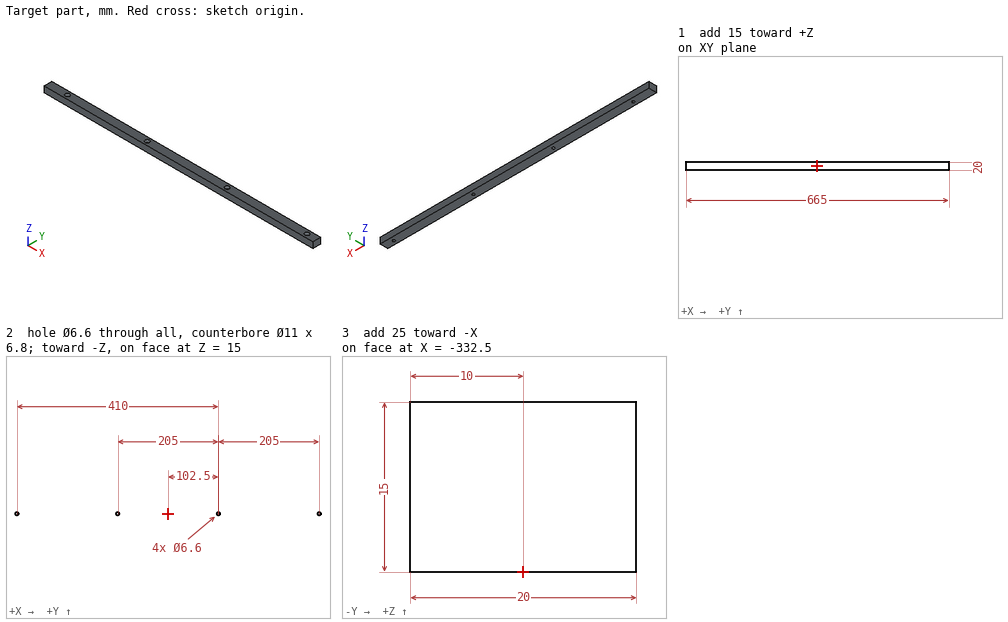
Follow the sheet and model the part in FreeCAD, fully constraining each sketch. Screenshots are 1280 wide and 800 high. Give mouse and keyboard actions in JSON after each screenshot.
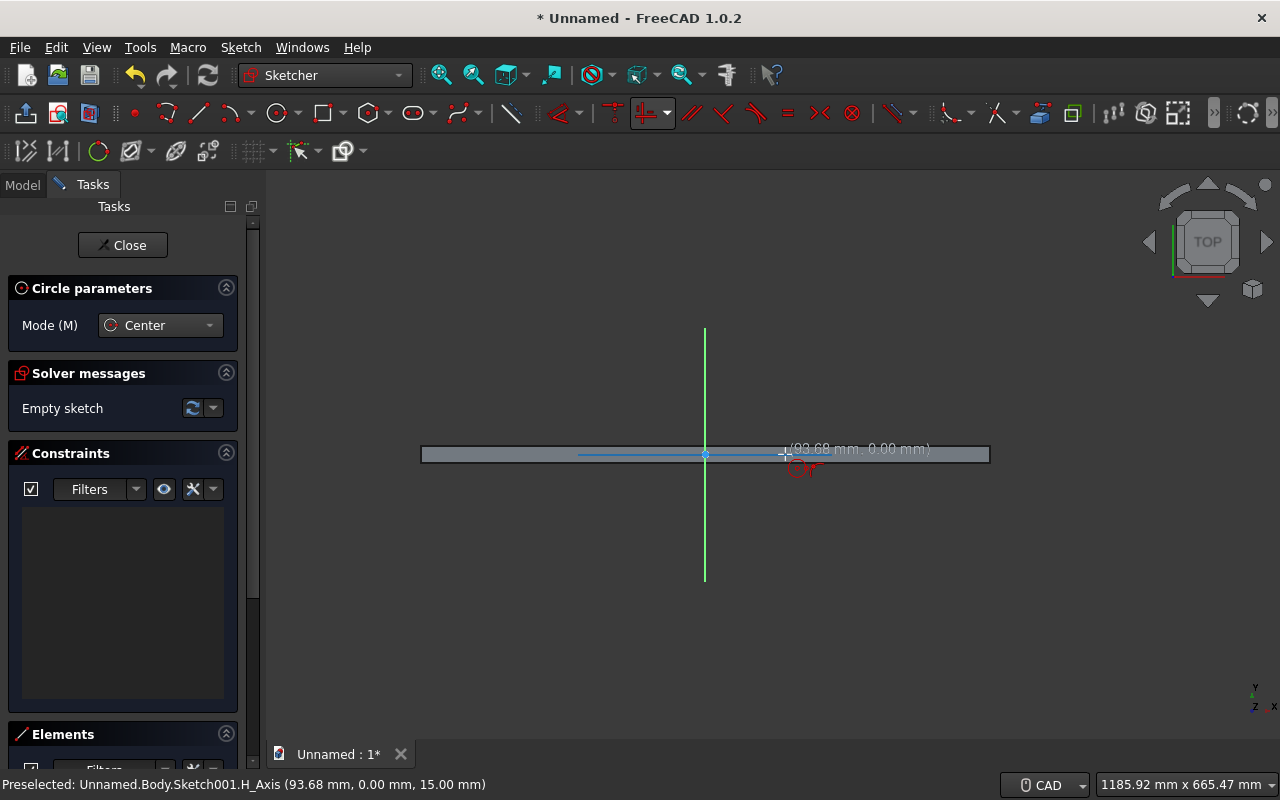
{"action": "left_click", "coordinate": [793, 454]}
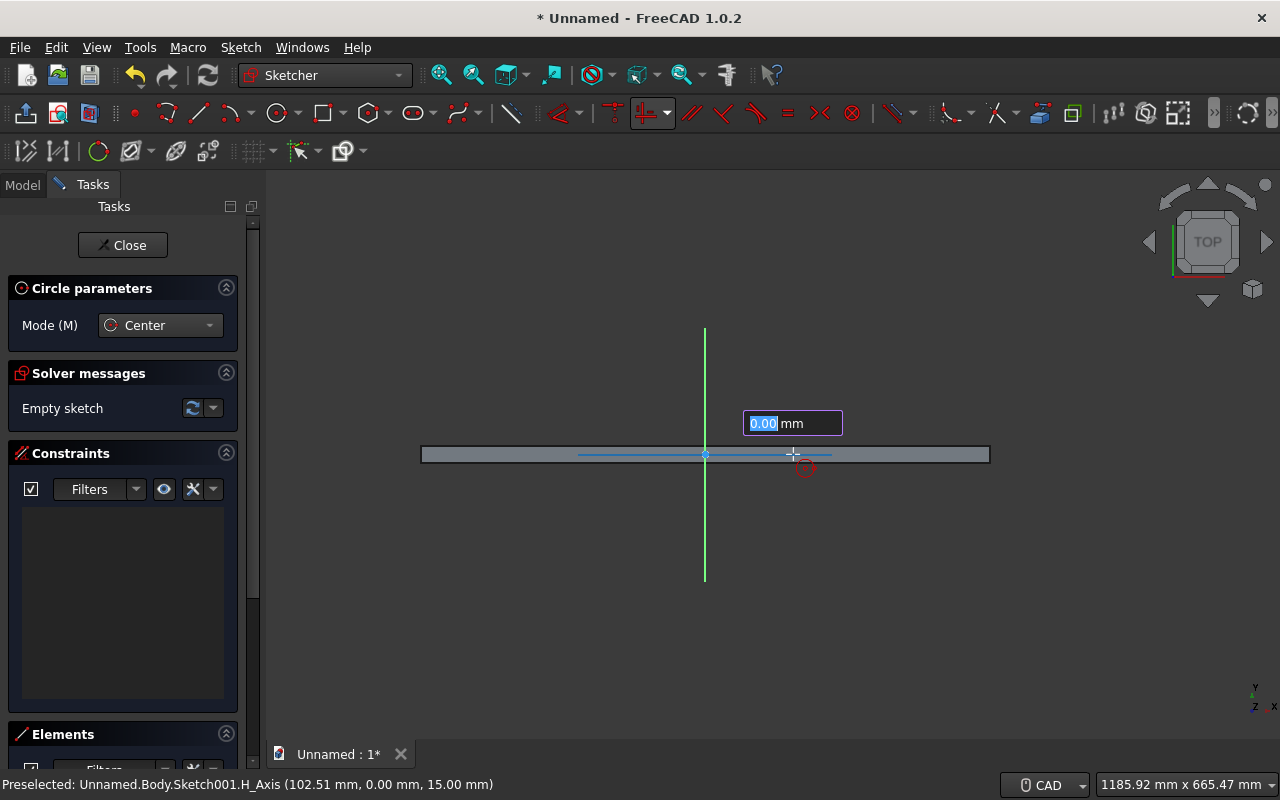
{"action": "scroll", "coordinate": [792, 457], "scroll_direction": "up", "scroll_amount": 9}
{"action": "mouse_move", "coordinate": [790, 455]}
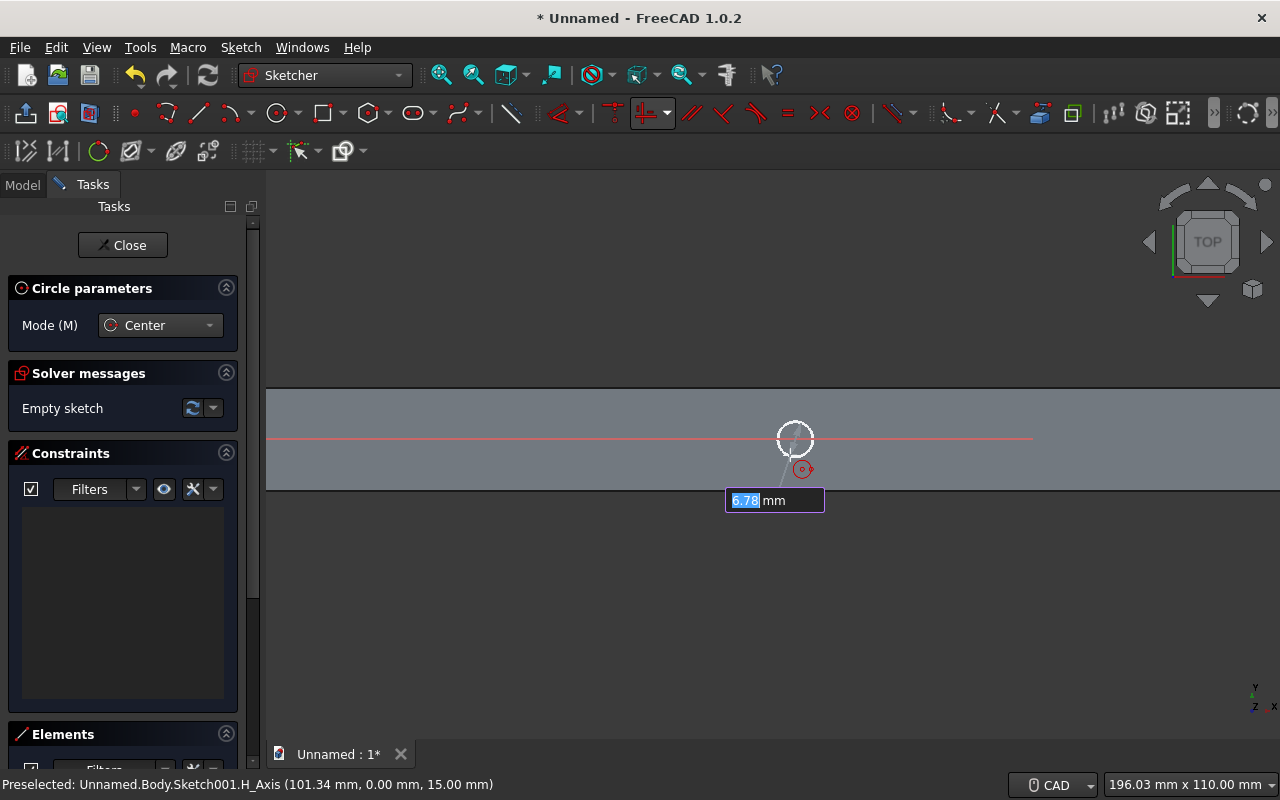
{"action": "type", "text": "6.6"}
{"action": "key", "text": "Return"}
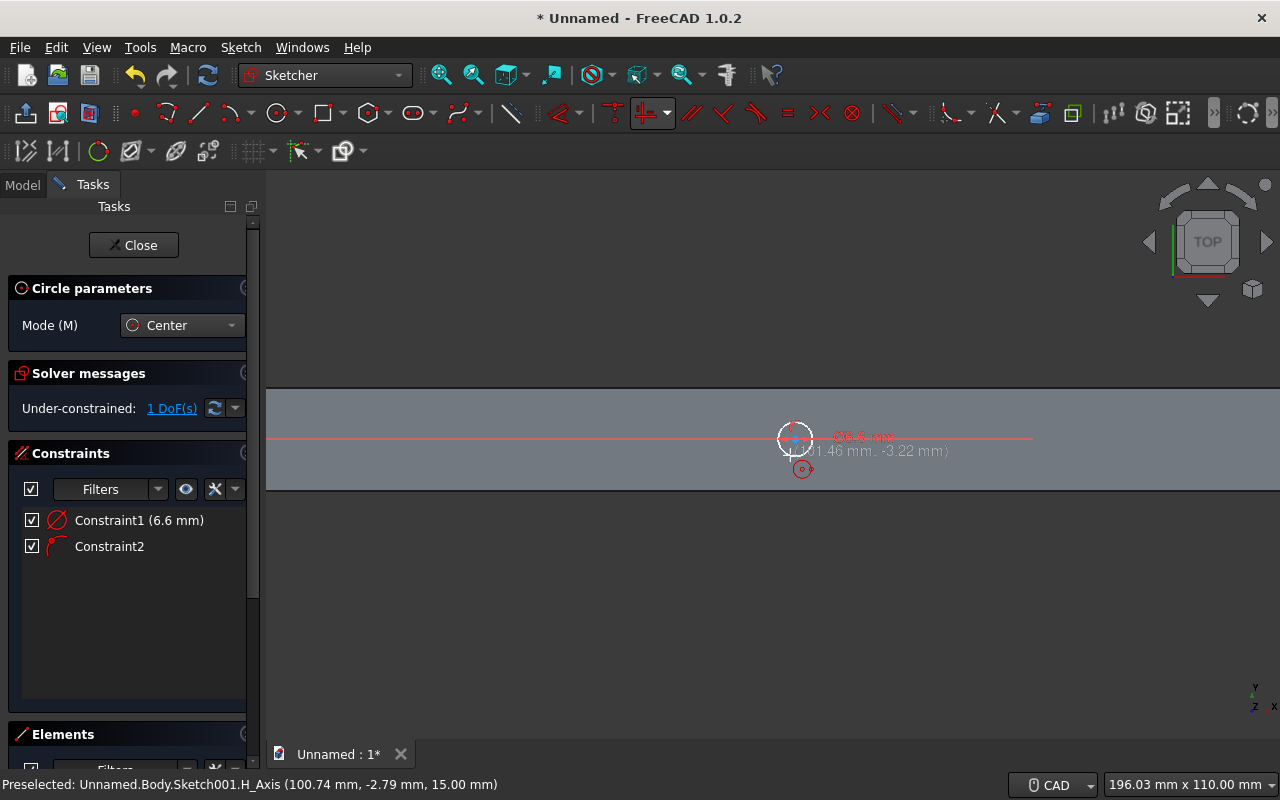
{"action": "scroll", "coordinate": [791, 458], "scroll_direction": "down", "scroll_amount": 9}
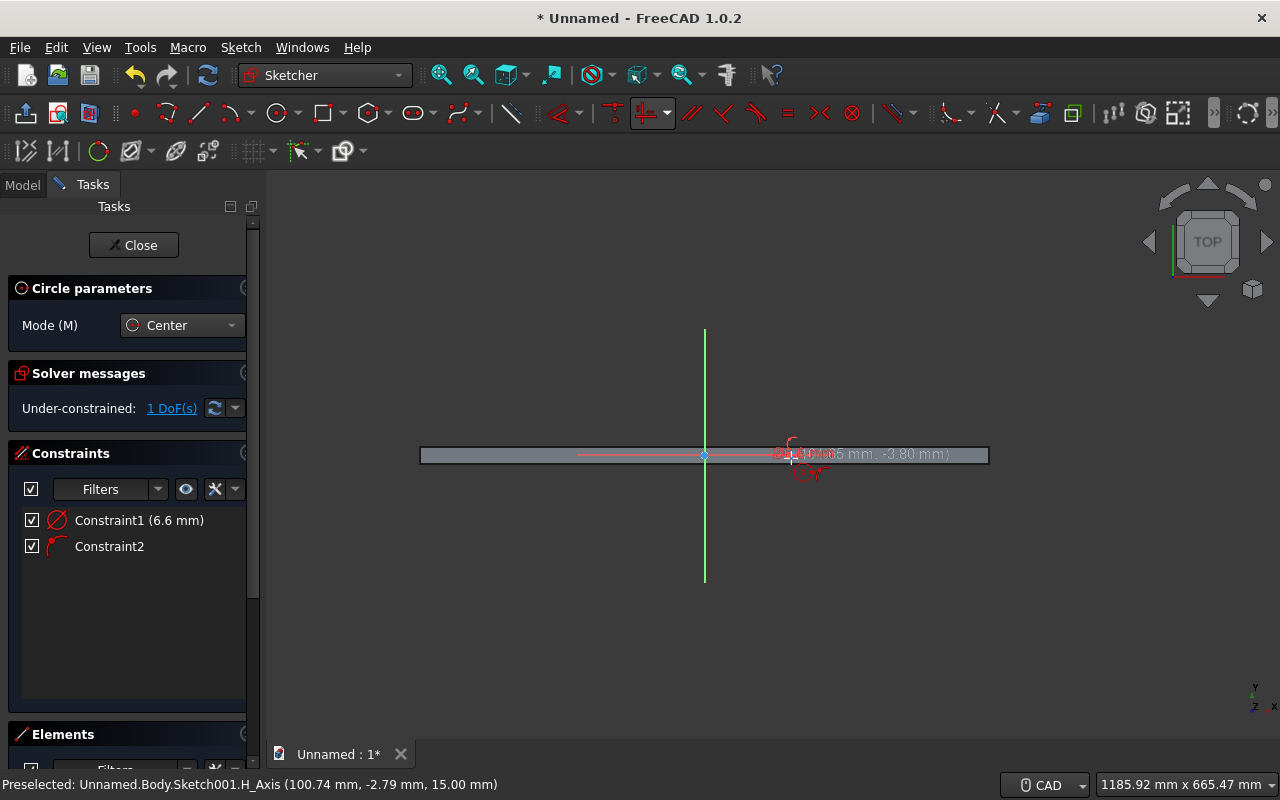
{"action": "scroll", "coordinate": [442, 455], "scroll_direction": "up", "scroll_amount": 11}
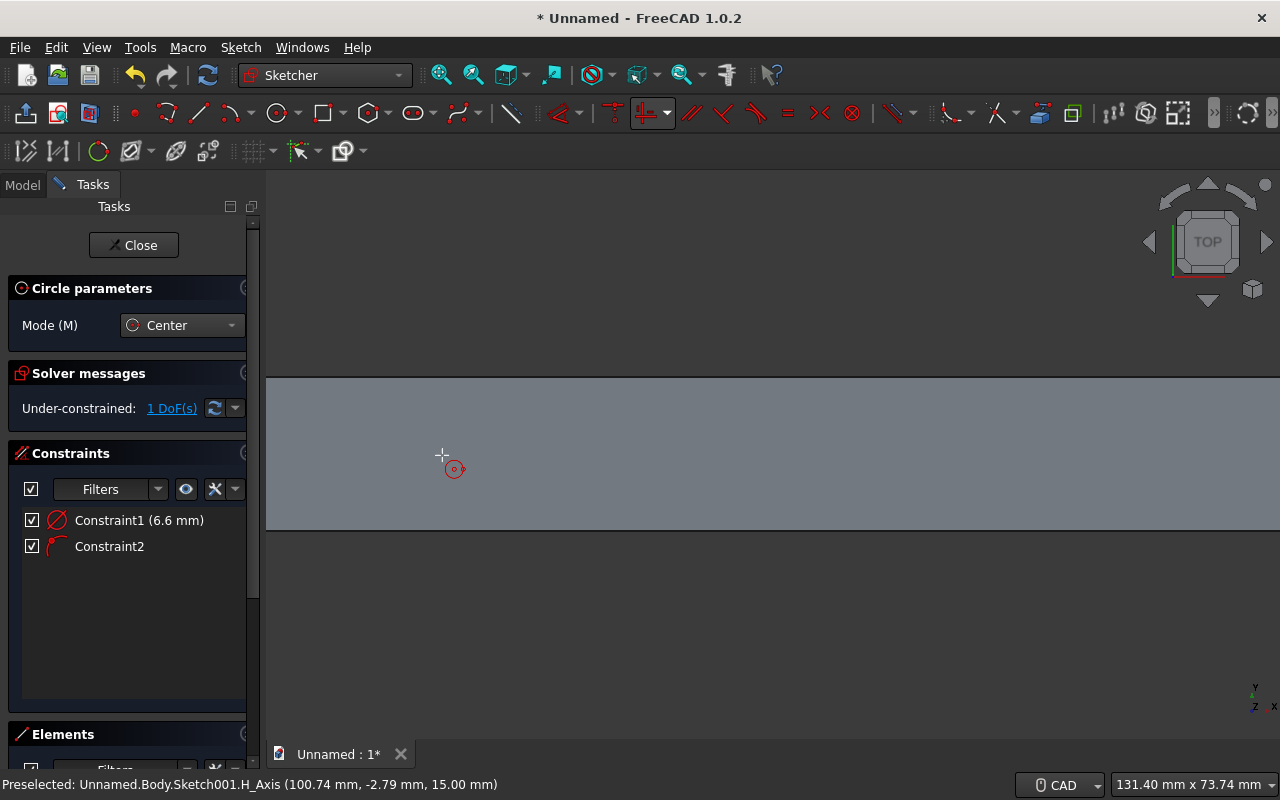
{"action": "scroll", "coordinate": [442, 455], "scroll_direction": "down", "scroll_amount": 11}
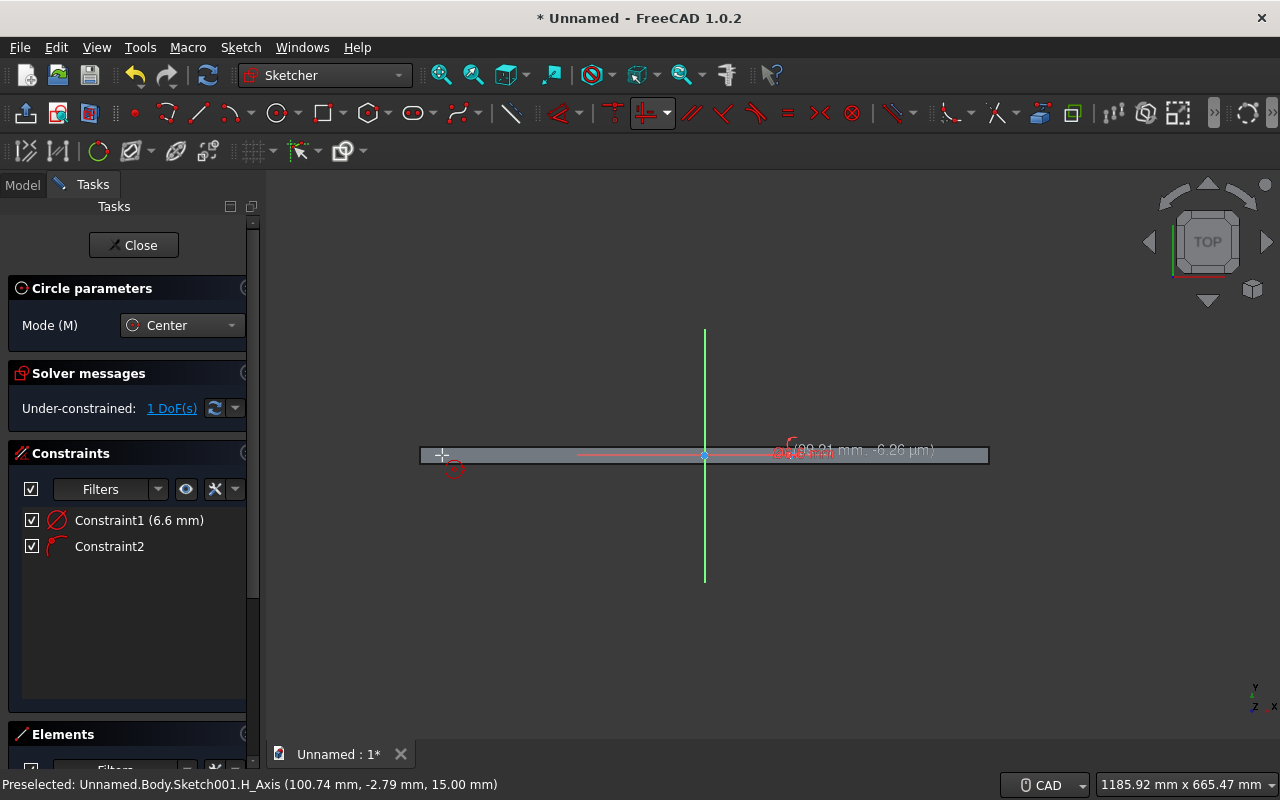
{"action": "left_click", "coordinate": [442, 455]}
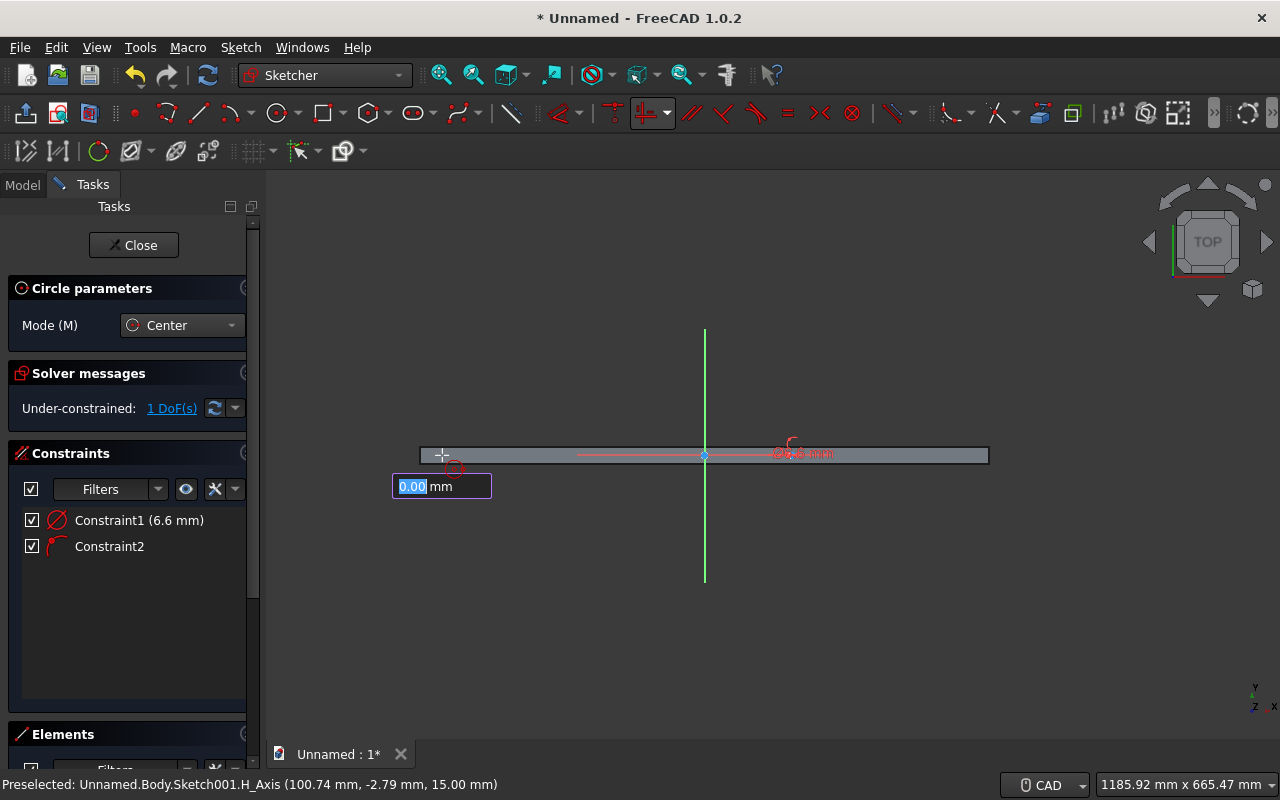
{"action": "scroll", "coordinate": [441, 458], "scroll_direction": "up", "scroll_amount": 9}
{"action": "mouse_move", "coordinate": [438, 455]}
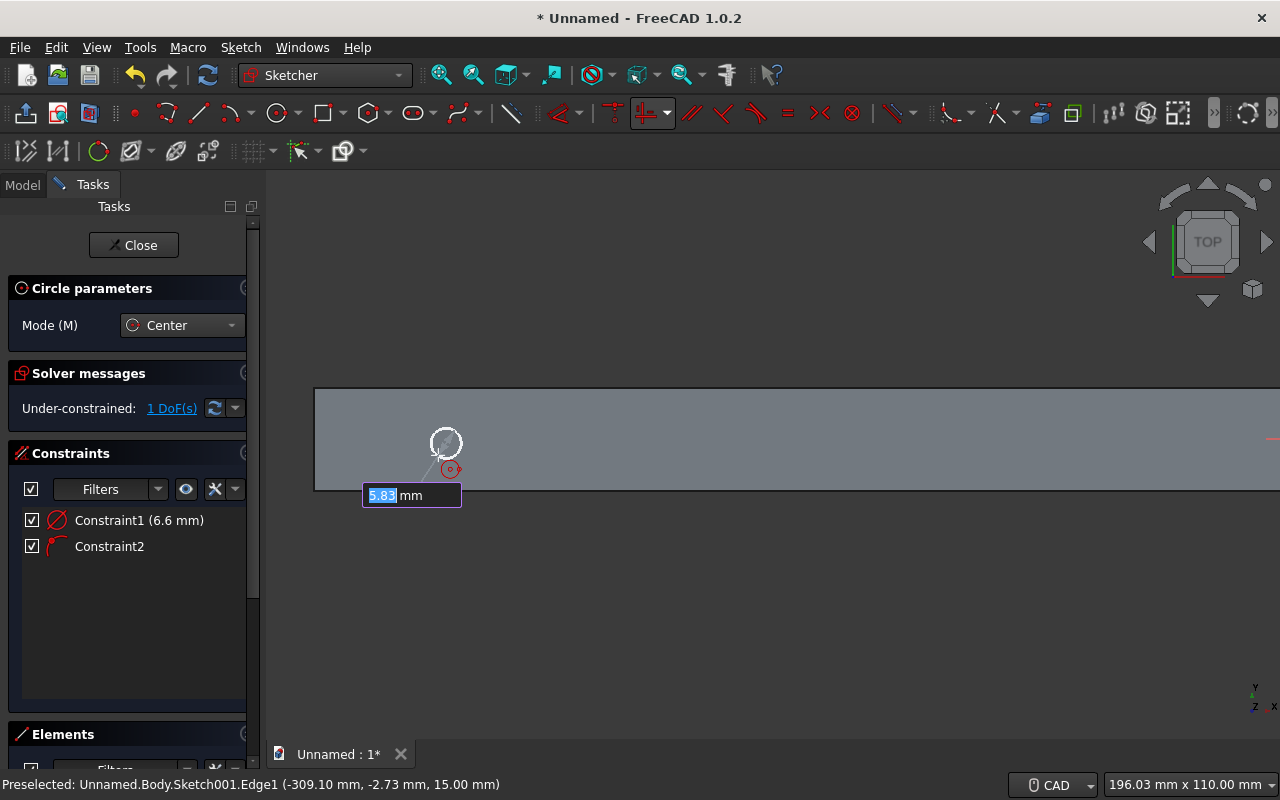
{"action": "type", "text": "6.6"}
{"action": "key", "text": "Return"}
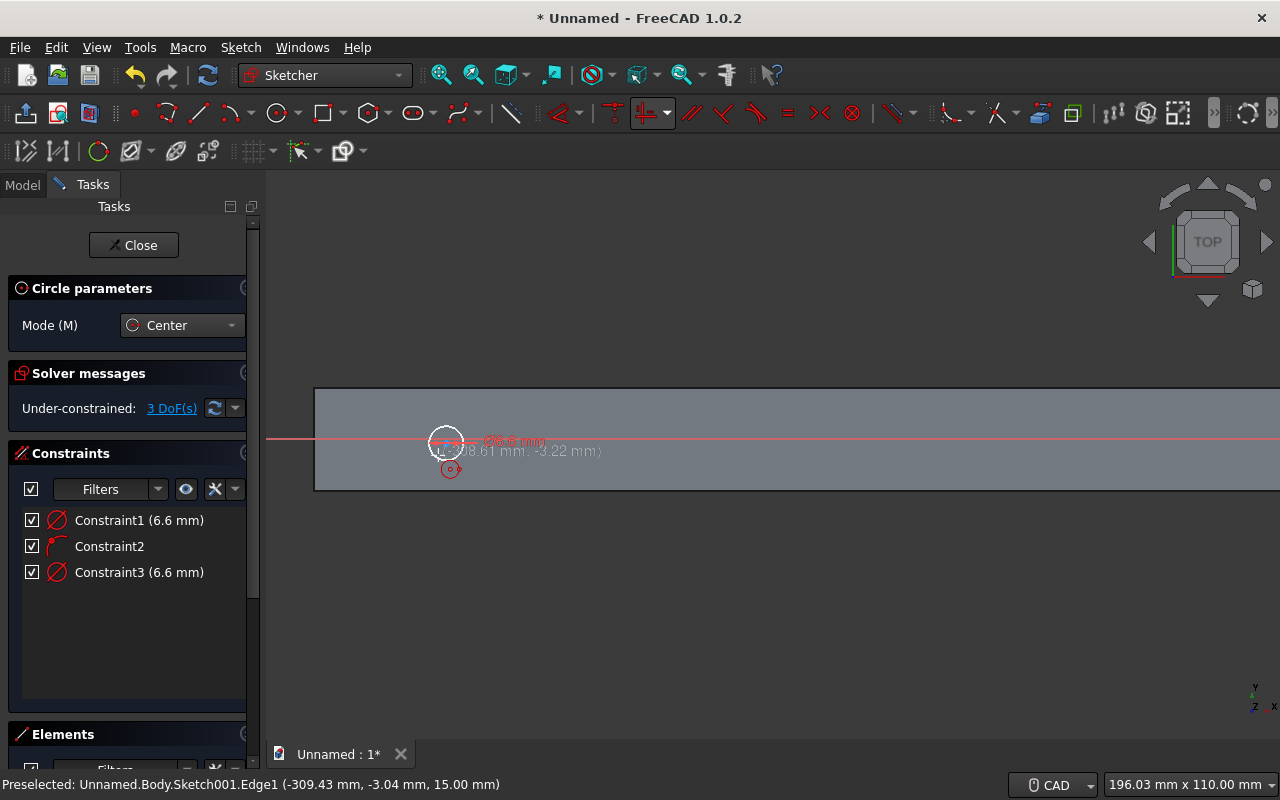
{"action": "scroll", "coordinate": [441, 458], "scroll_direction": "down", "scroll_amount": 9}